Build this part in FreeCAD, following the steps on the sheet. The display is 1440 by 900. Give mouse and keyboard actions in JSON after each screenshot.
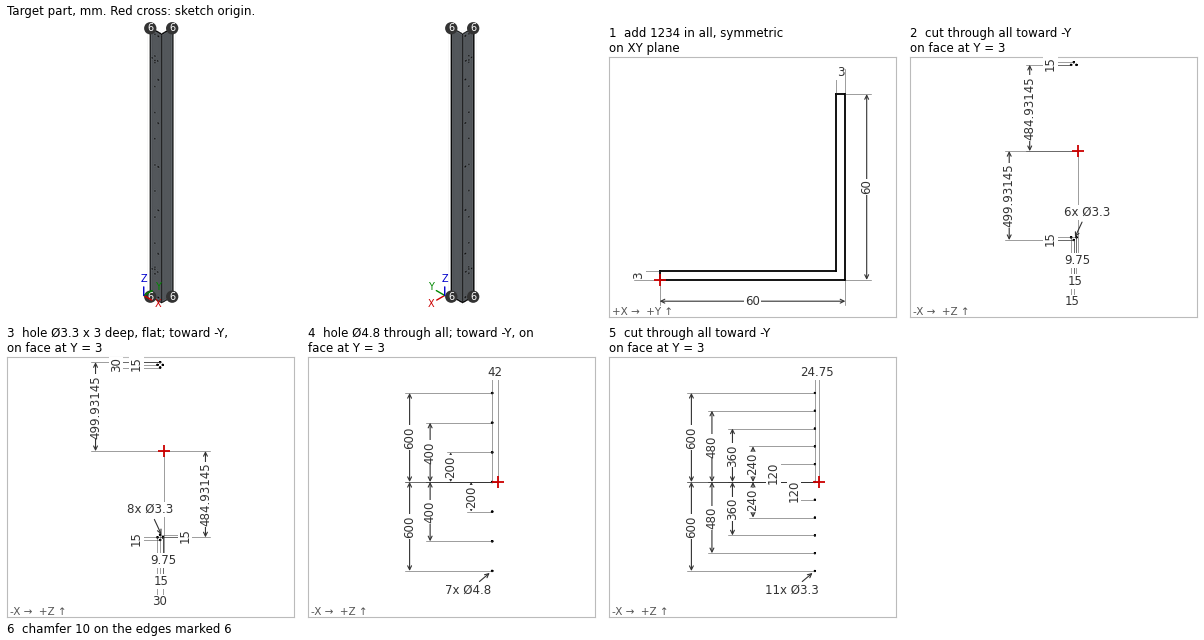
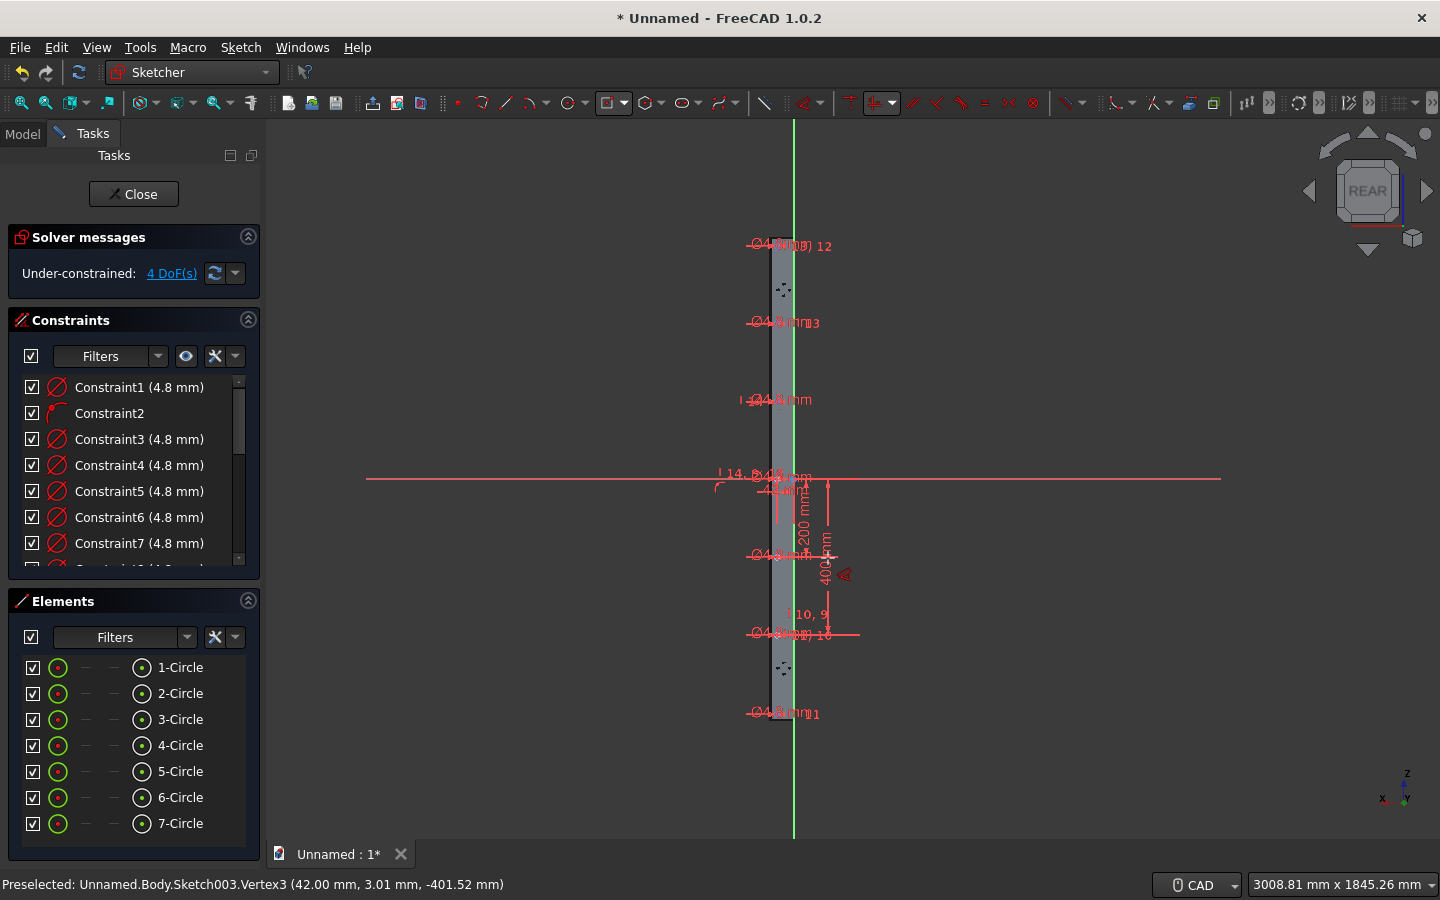
{"action": "left_click", "coordinate": [777, 714]}
{"action": "left_click", "coordinate": [828, 597]}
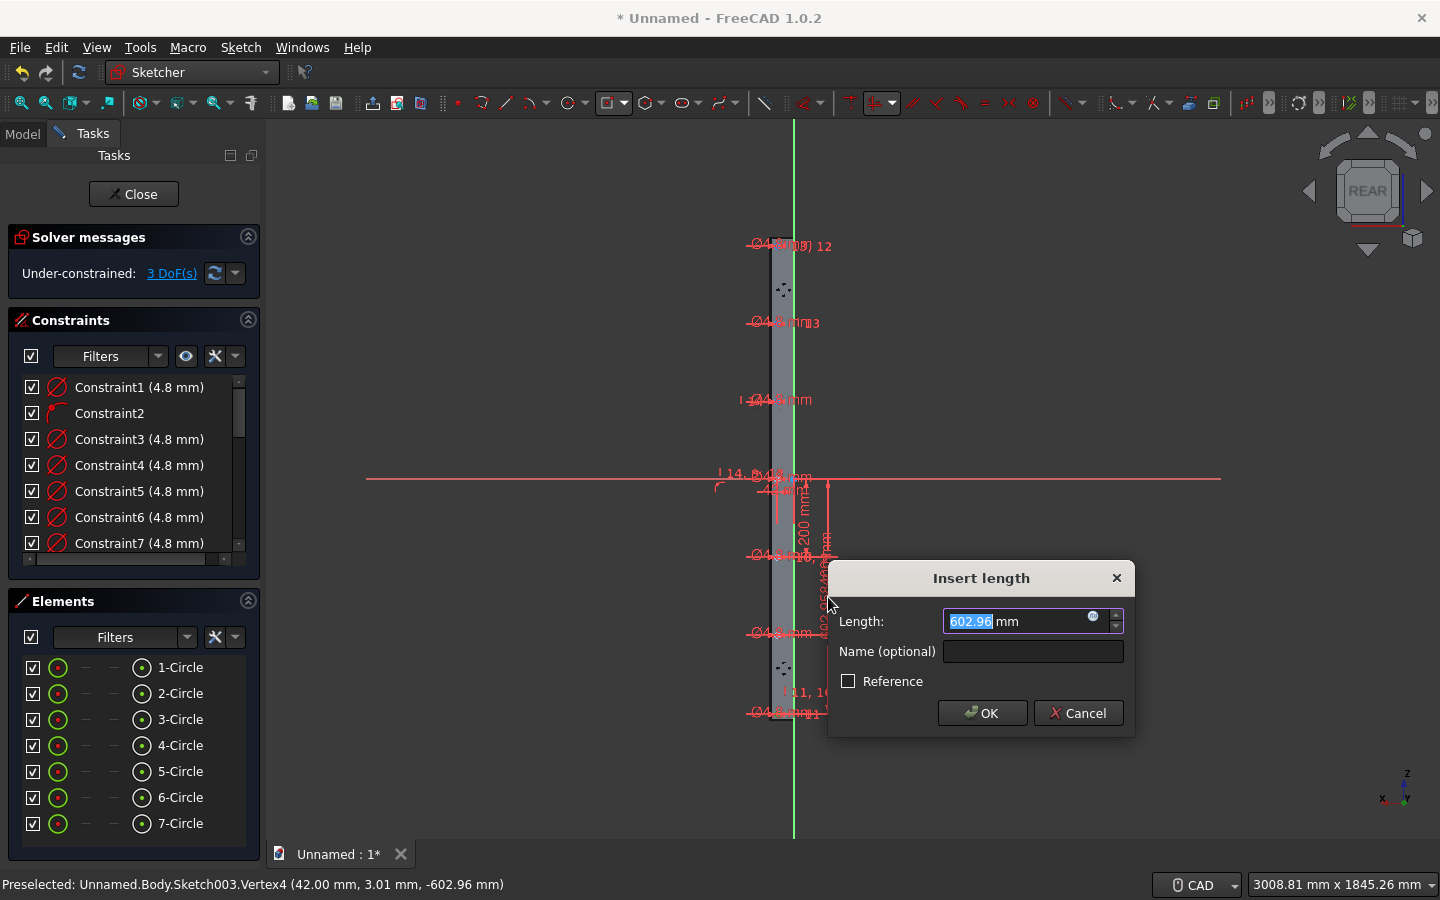
{"action": "type", "text": "600"}
{"action": "key", "text": "Return"}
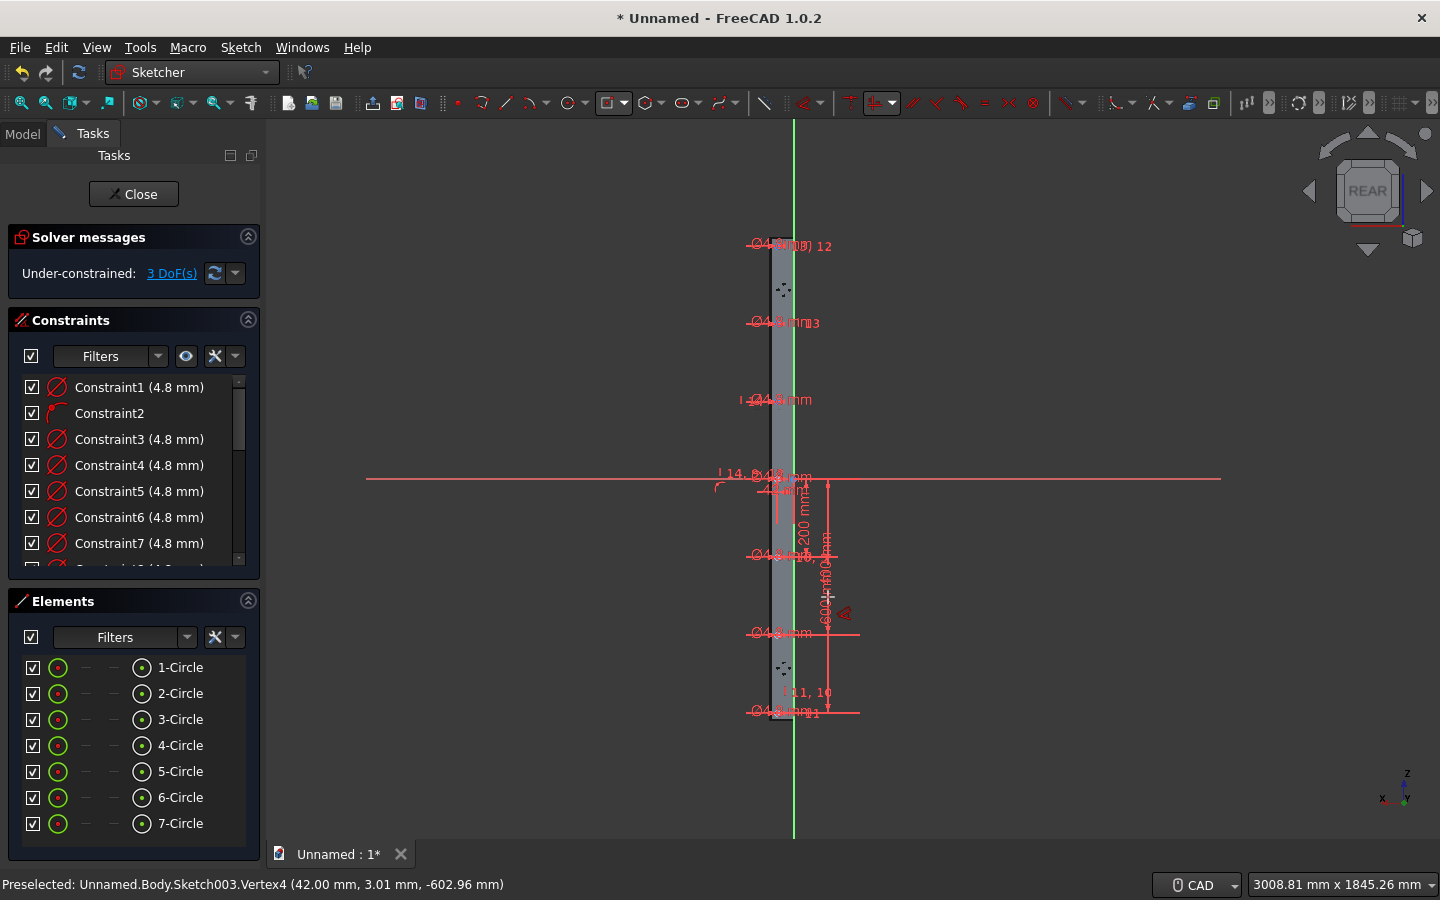
{"action": "left_click", "coordinate": [777, 246]}
{"action": "left_click", "coordinate": [828, 363]}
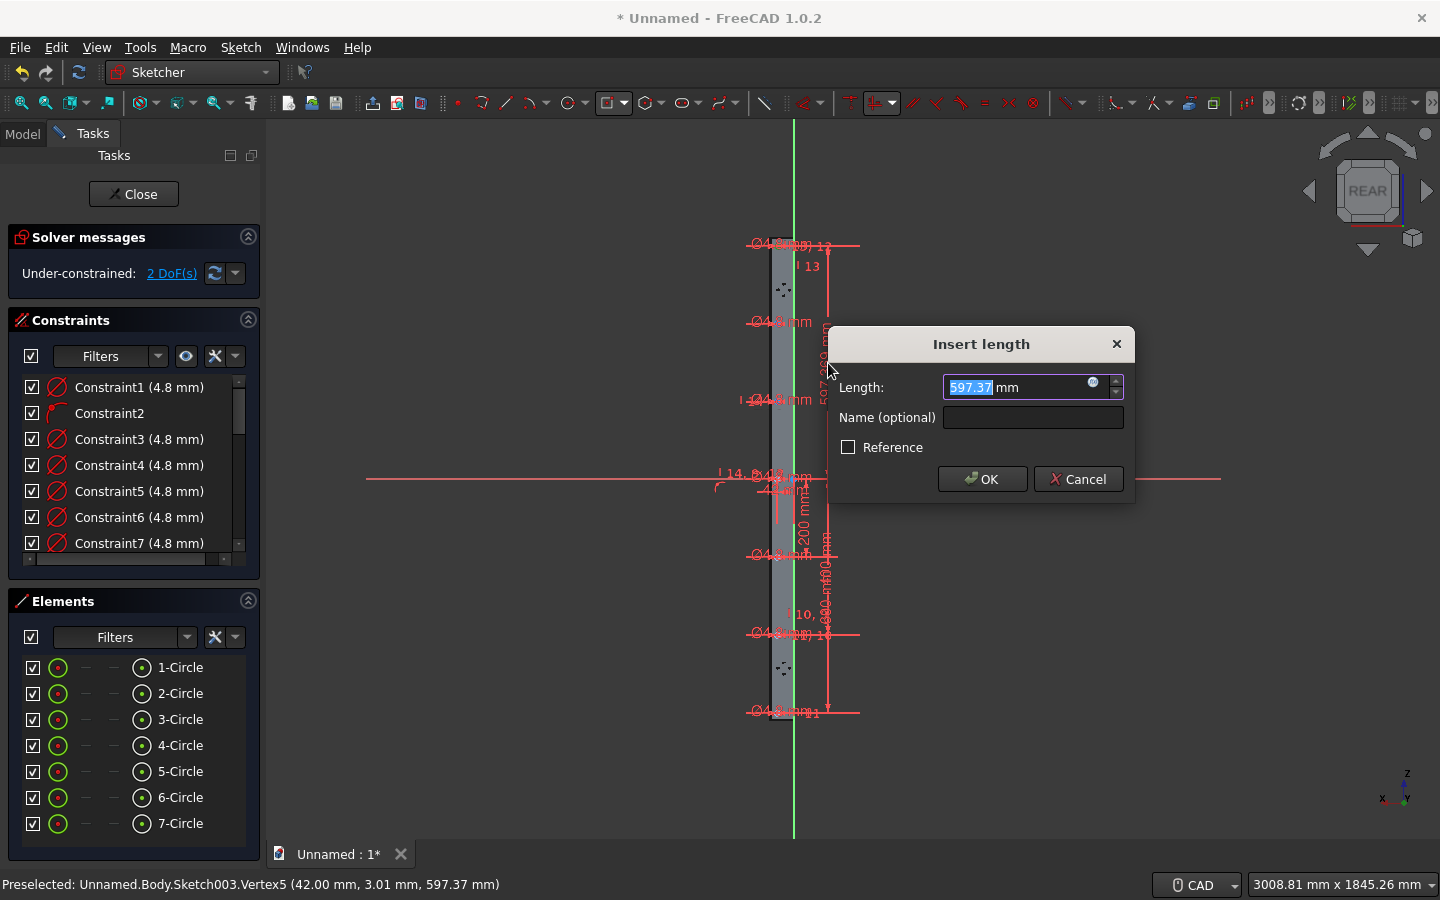
{"action": "type", "text": "600"}
{"action": "key", "text": "Return"}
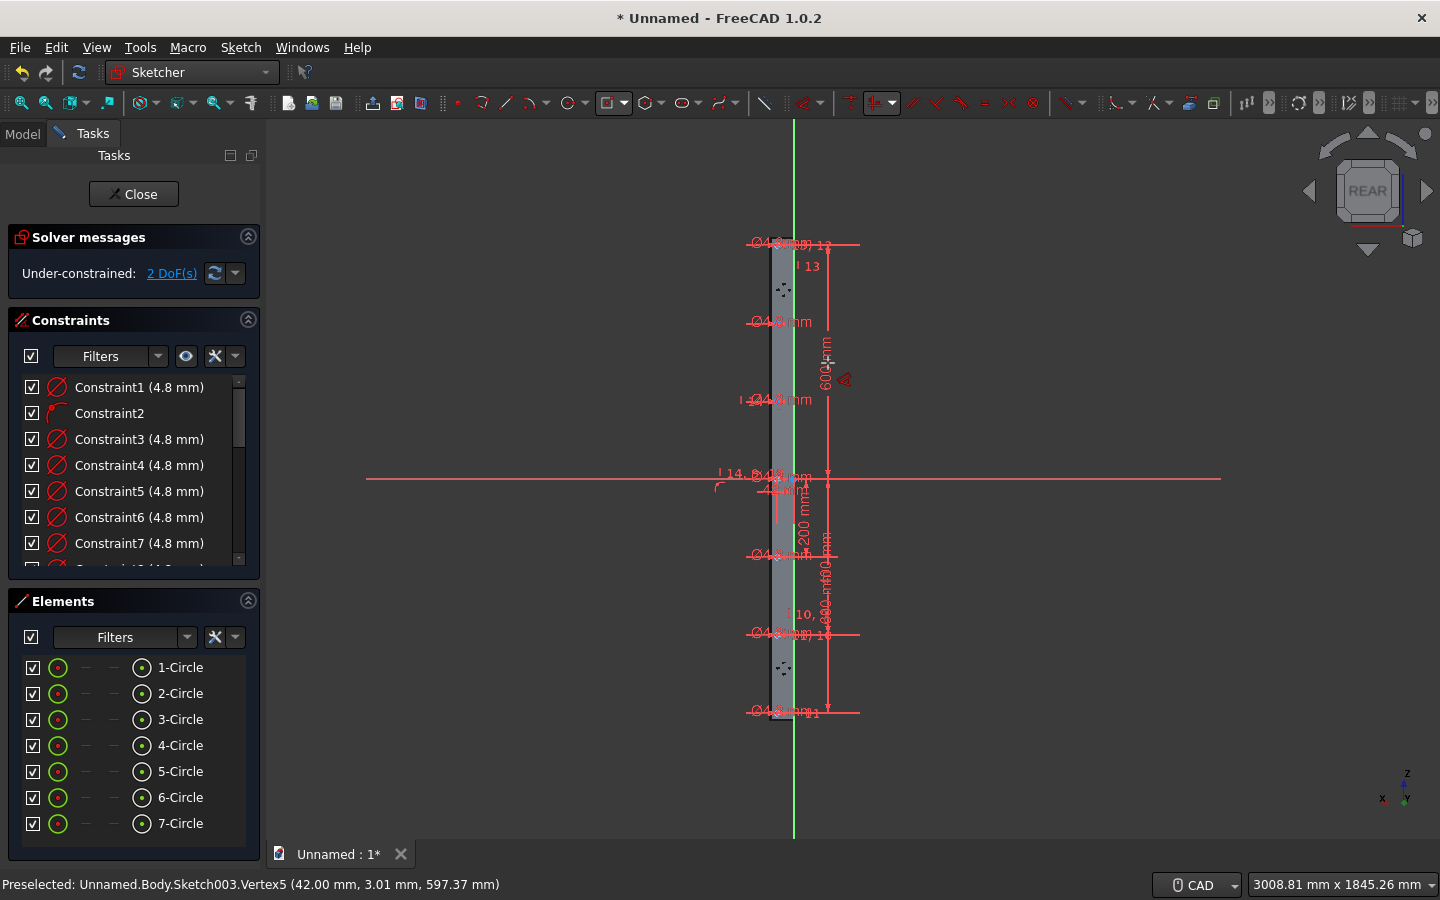
{"action": "left_click", "coordinate": [777, 324]}
{"action": "left_click", "coordinate": [828, 402]}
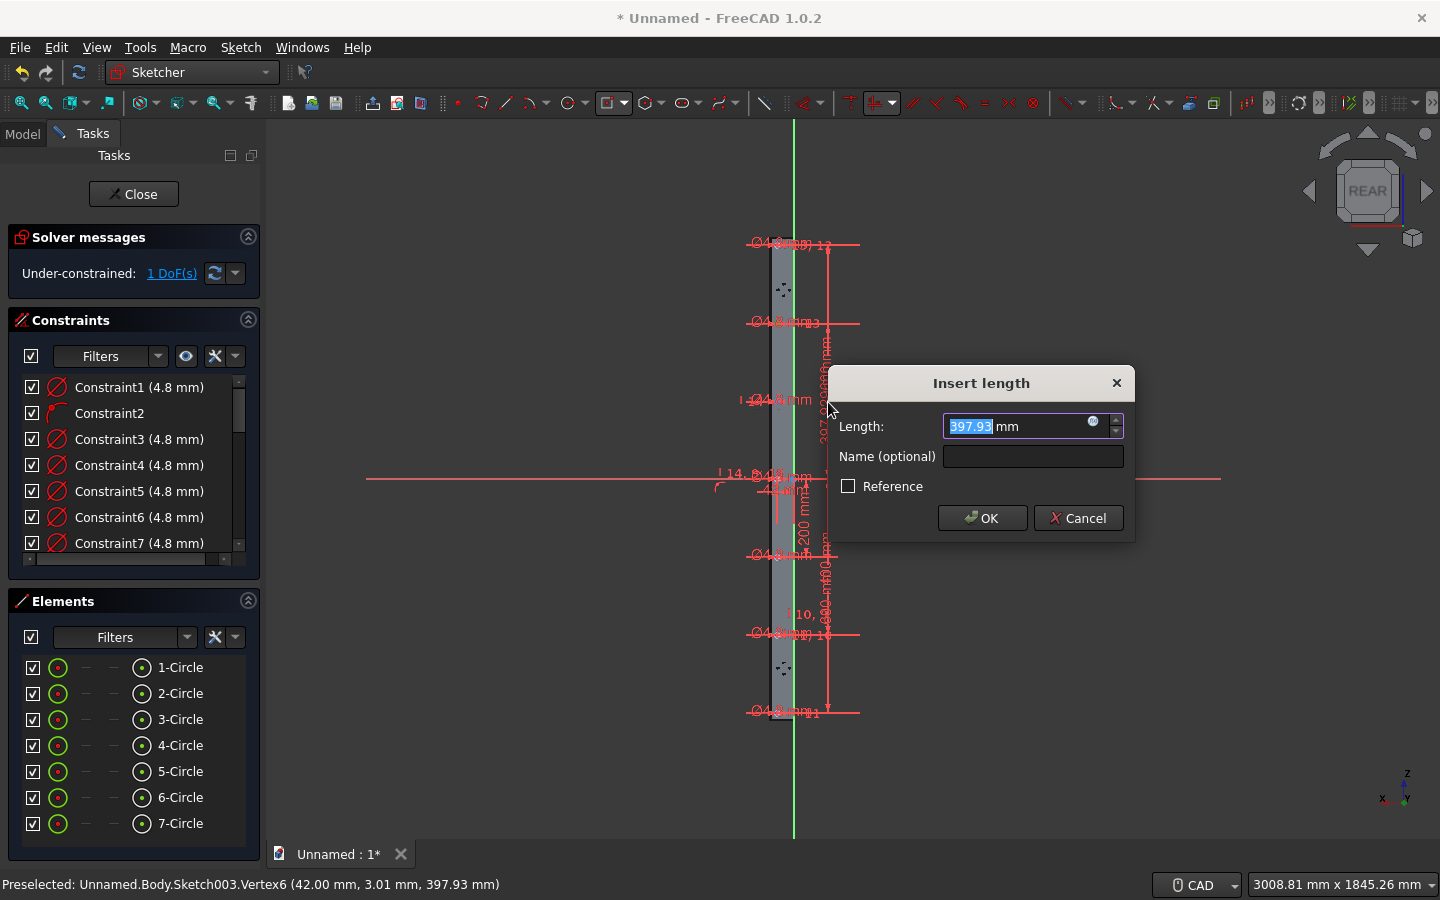
{"action": "type", "text": "400"}
{"action": "key", "text": "Return"}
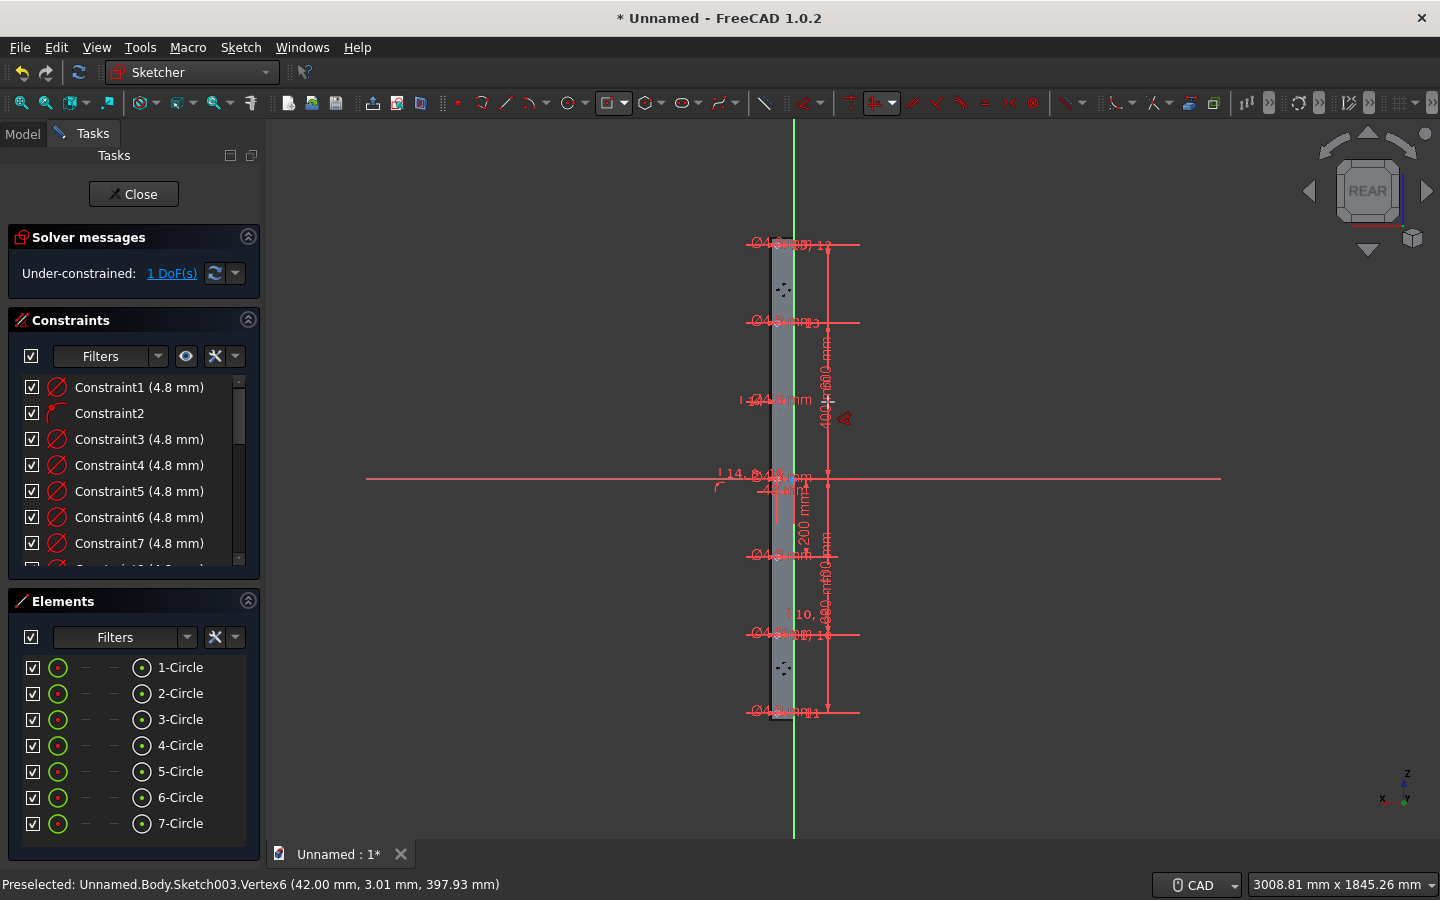
{"action": "left_click", "coordinate": [777, 402]}
{"action": "left_click", "coordinate": [828, 440]}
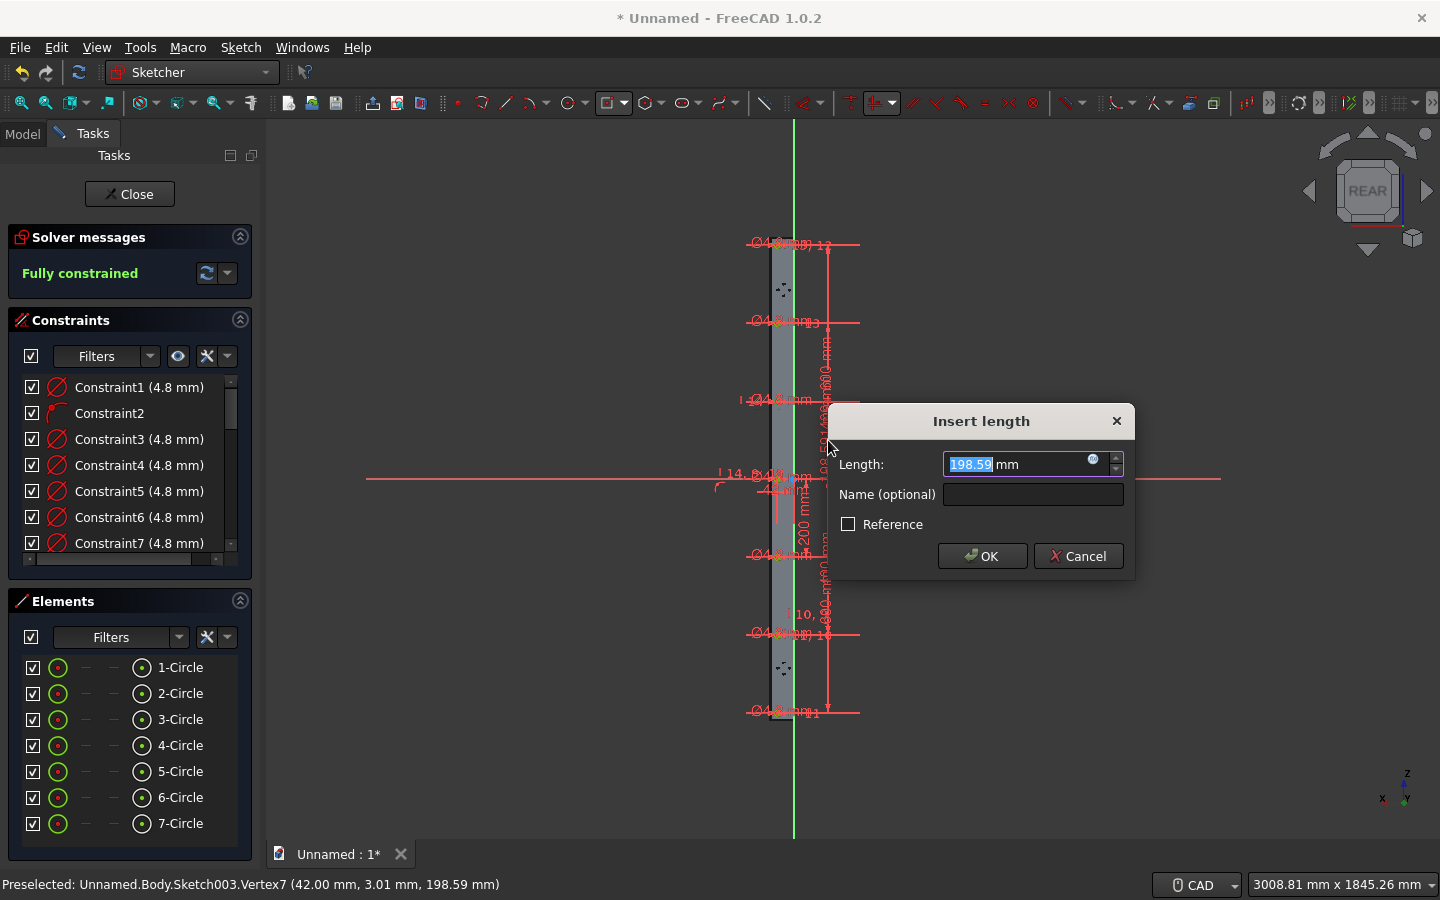
{"action": "type", "text": "200"}
{"action": "key", "text": "Return"}
{"action": "key", "text": "Escape"}